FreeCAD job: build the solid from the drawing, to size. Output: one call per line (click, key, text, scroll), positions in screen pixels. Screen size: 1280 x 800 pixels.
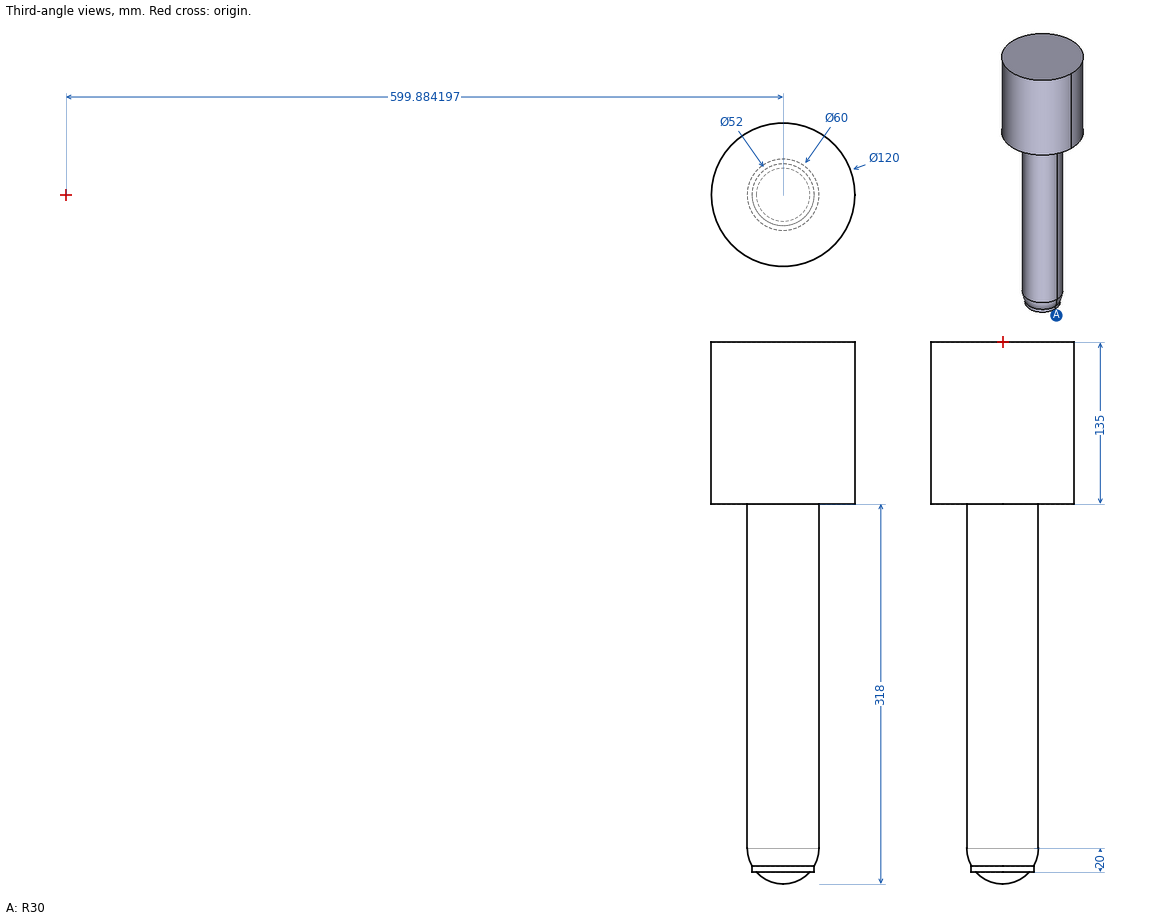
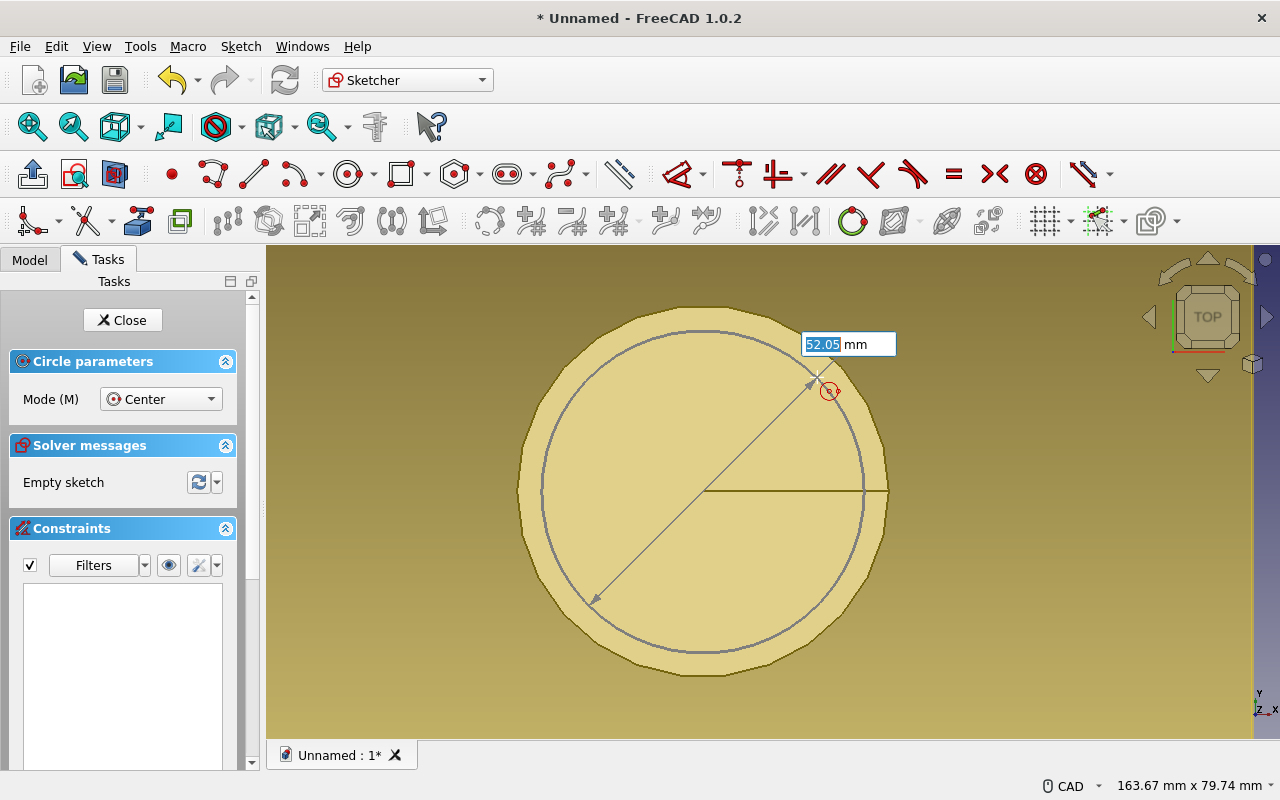
text(52)
key(Return)
key(Escape)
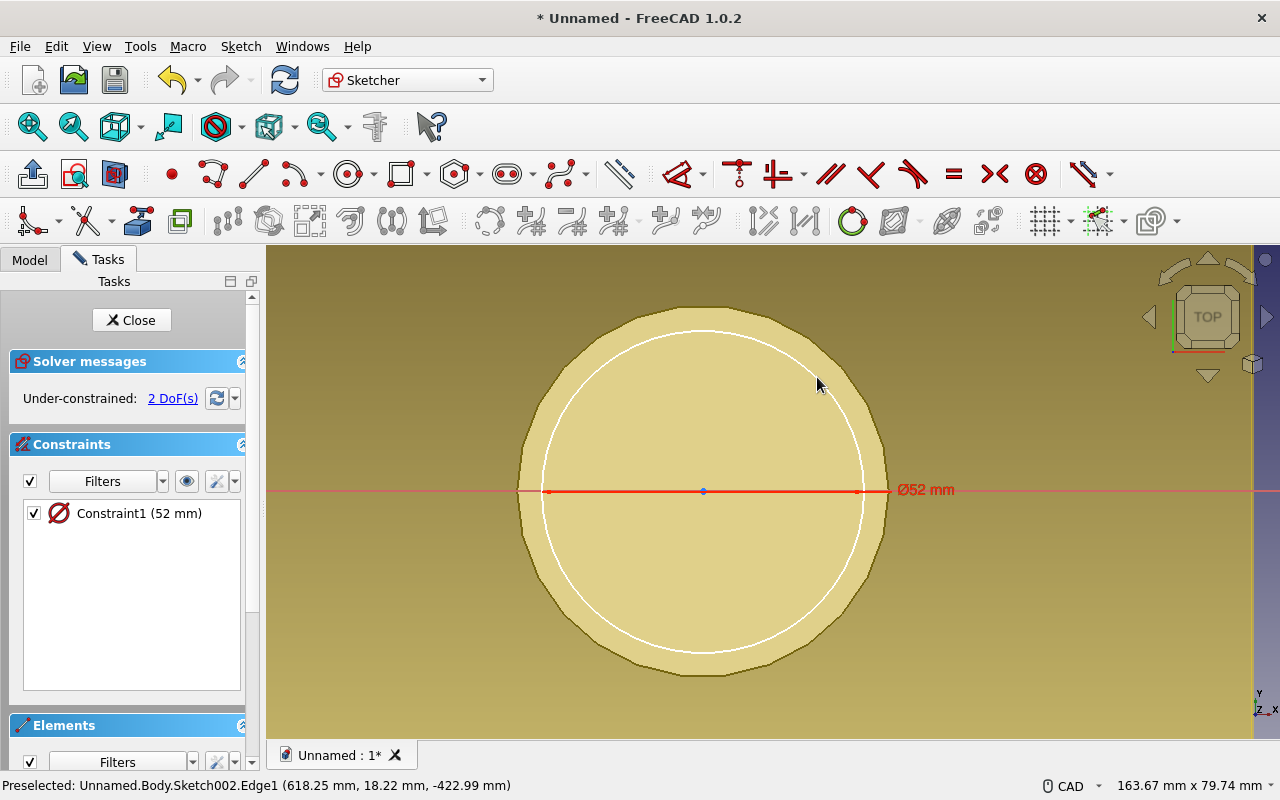
click(703, 492)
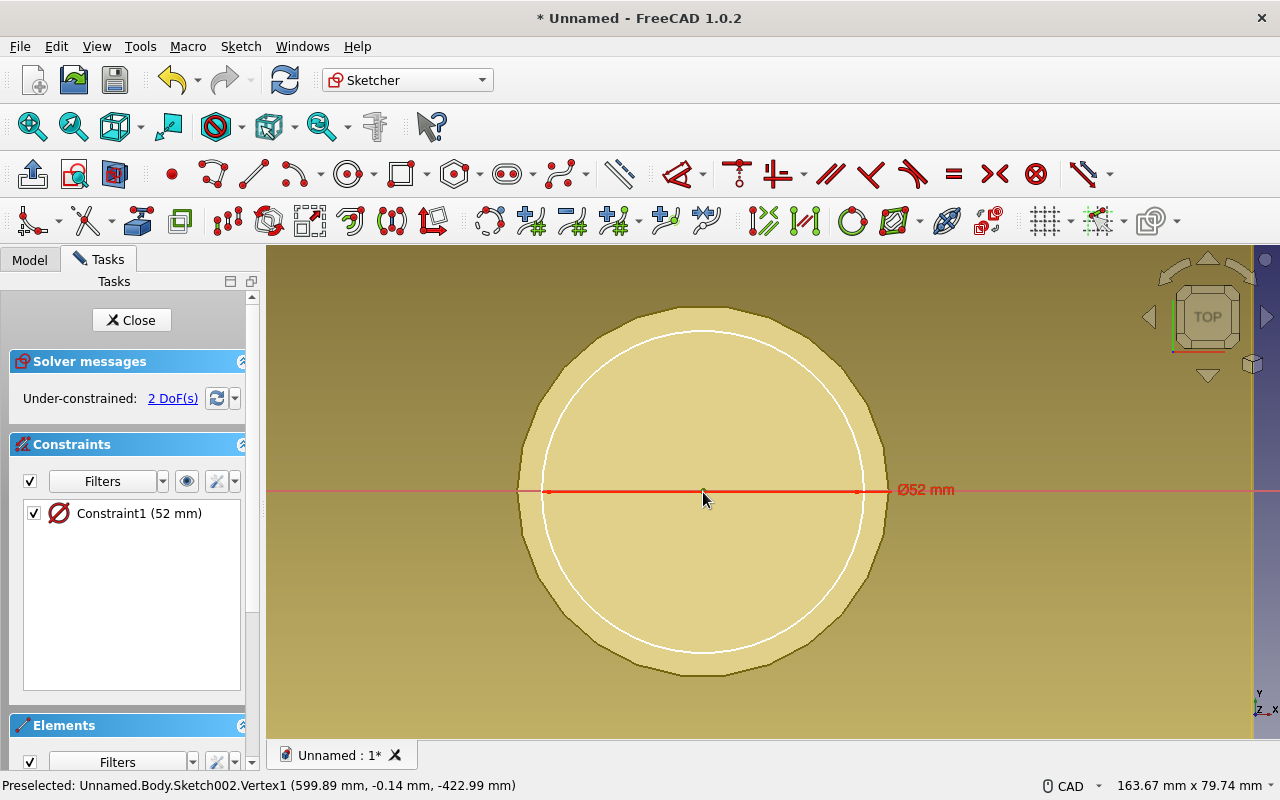
click(353, 491)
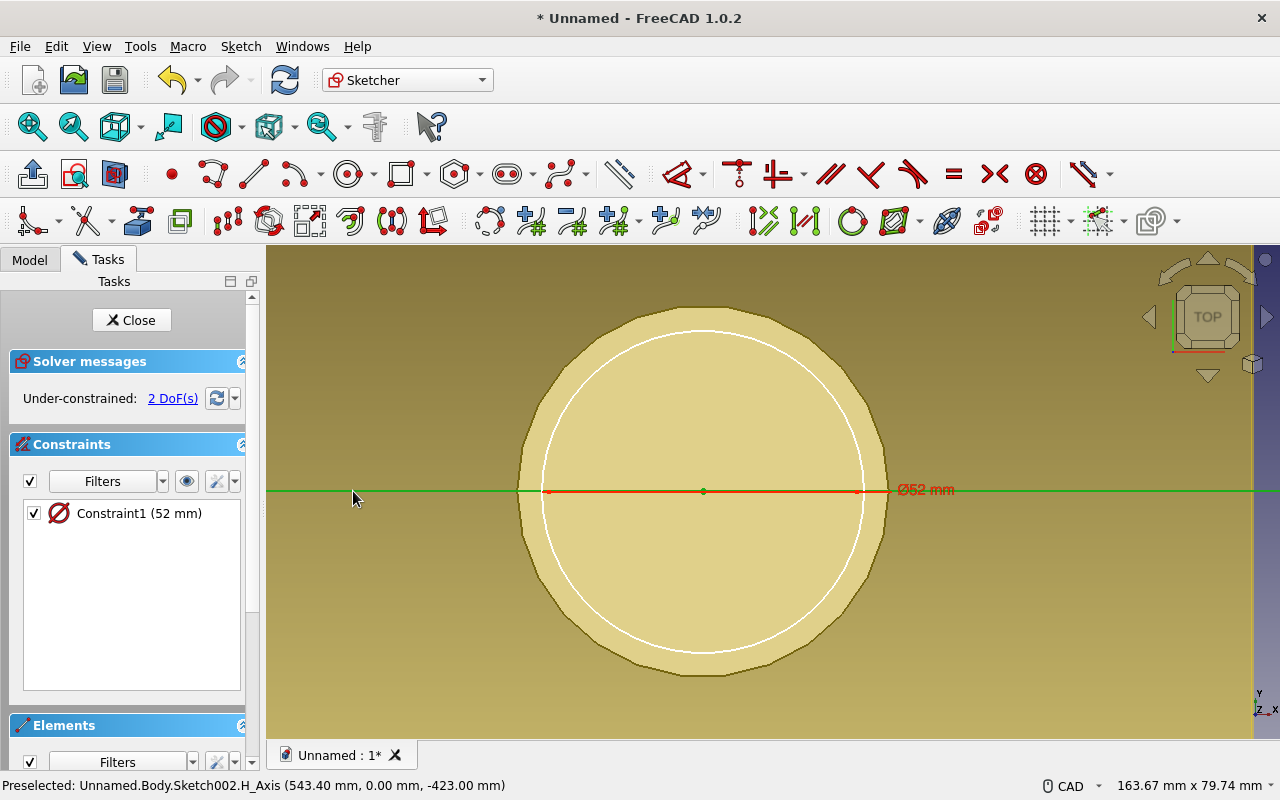
click(737, 174)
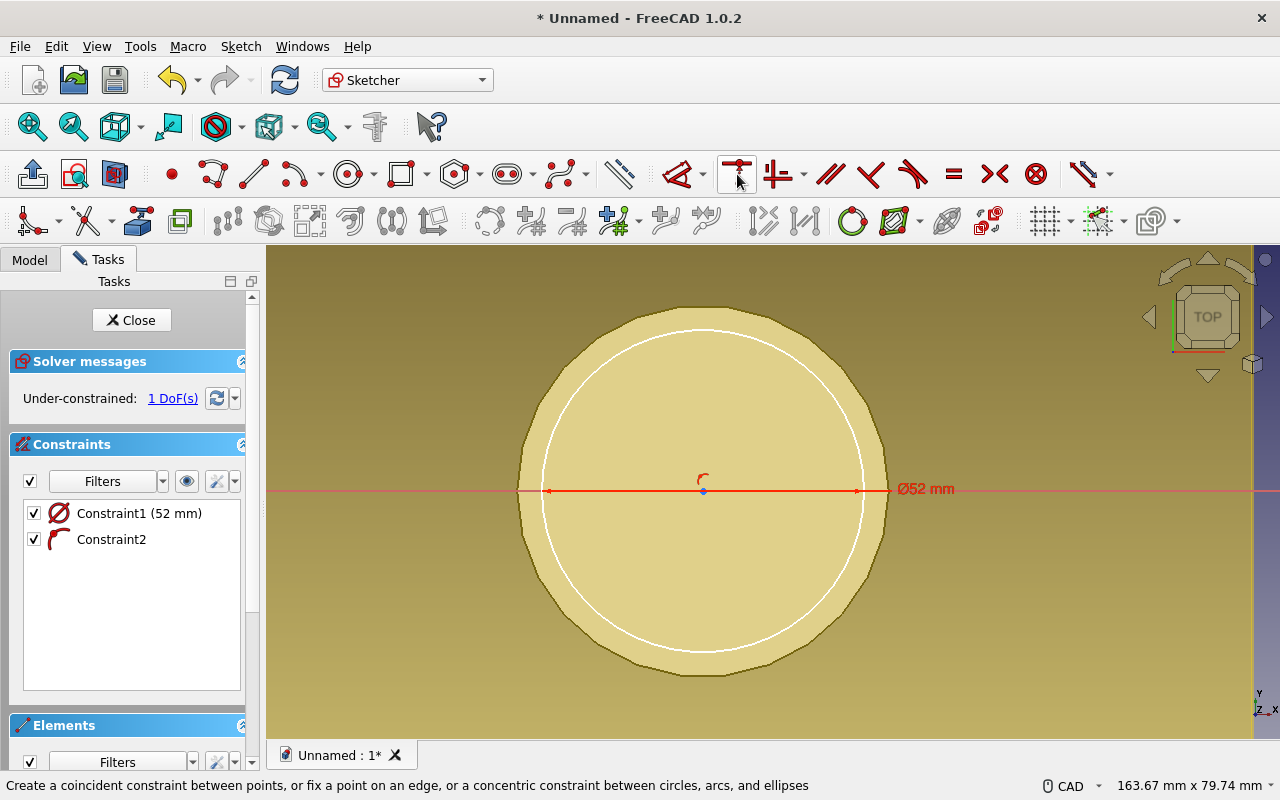
click(676, 174)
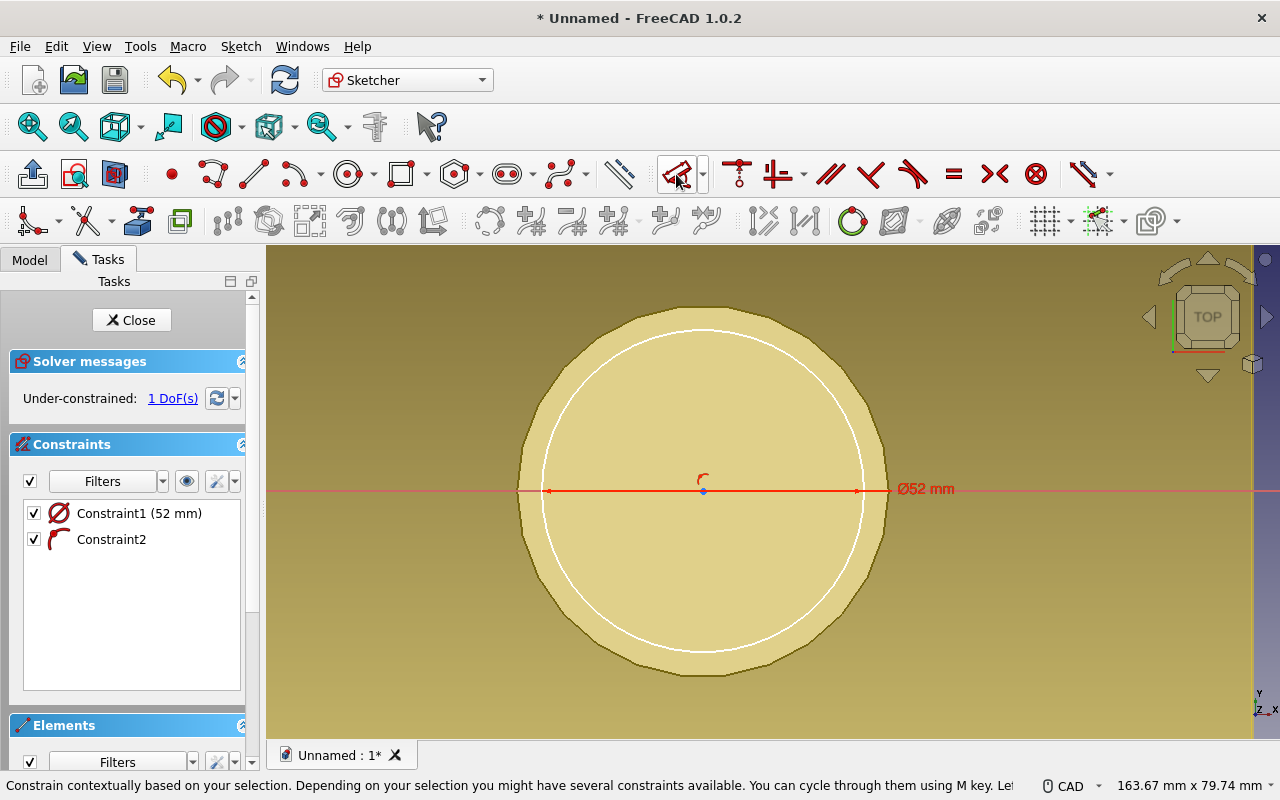
click(703, 491)
click(499, 525)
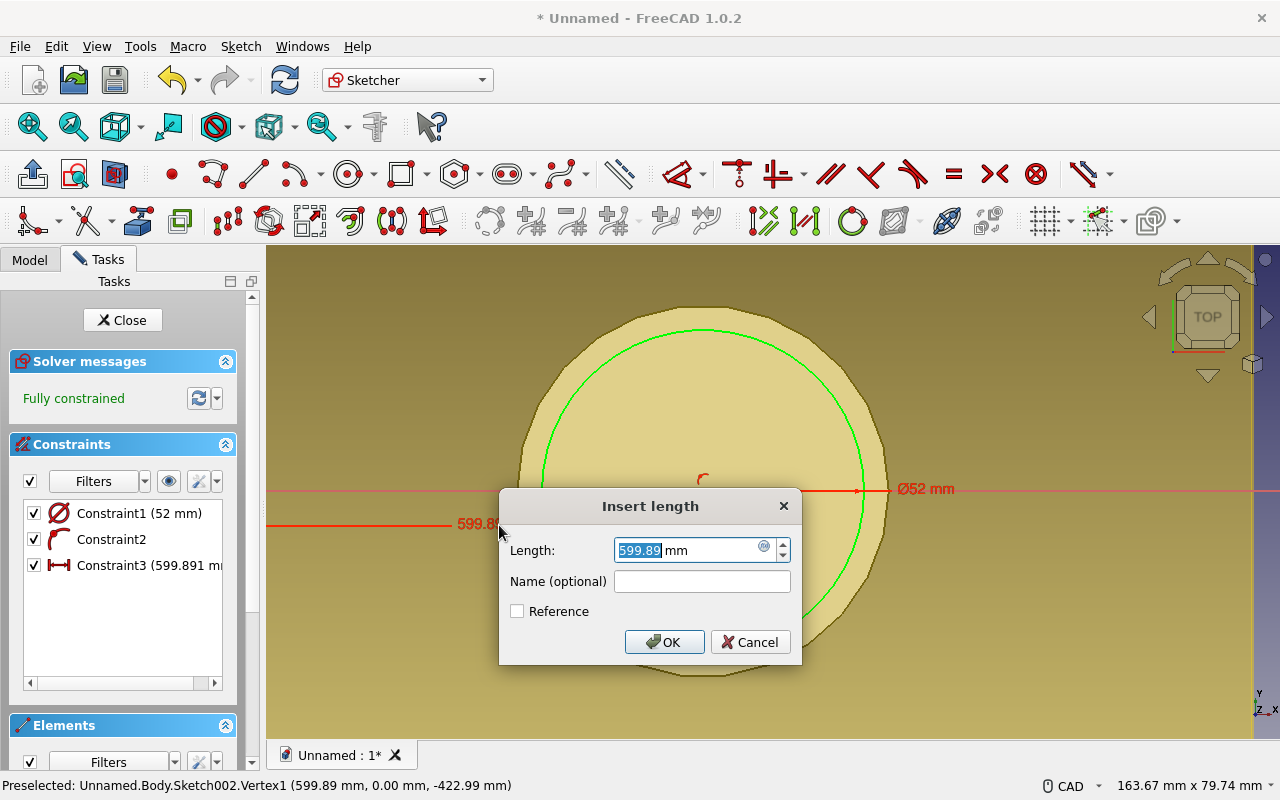
text(599.884197)
key(Return)
key(Escape)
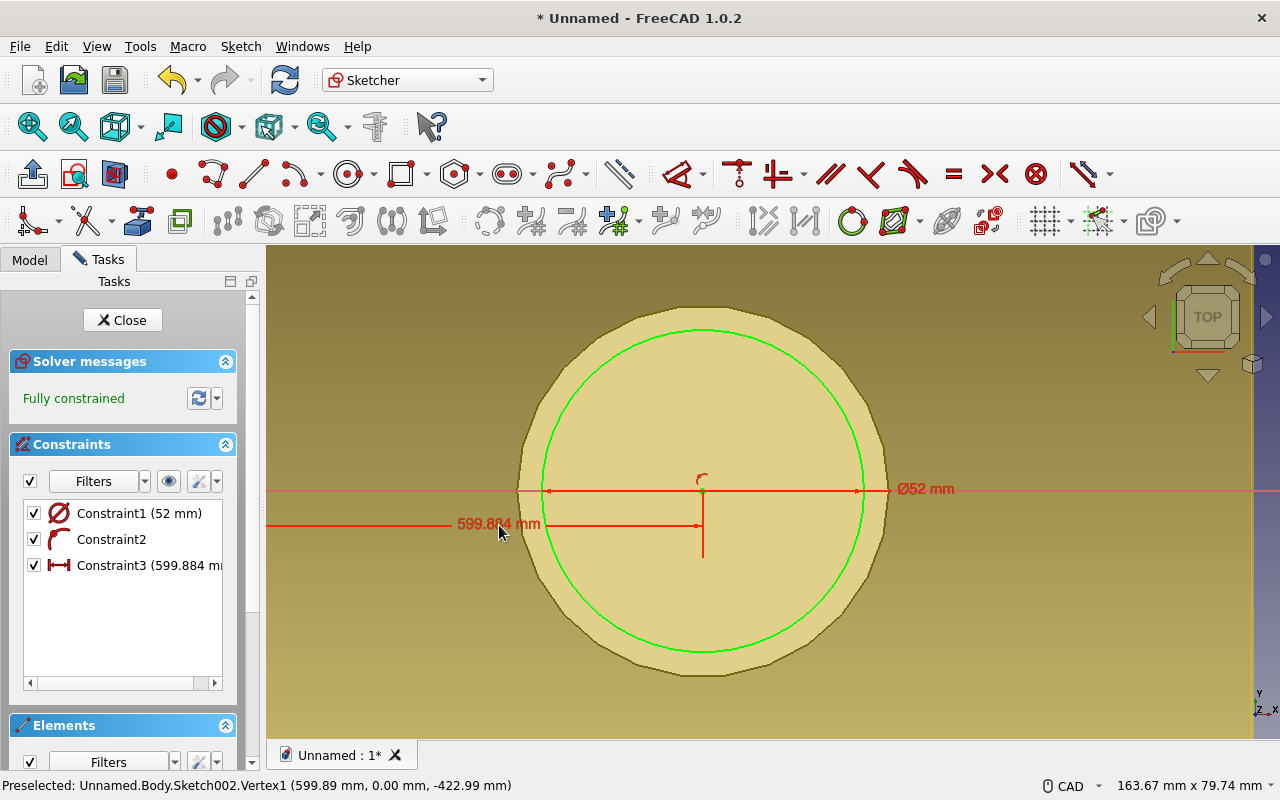
click(123, 320)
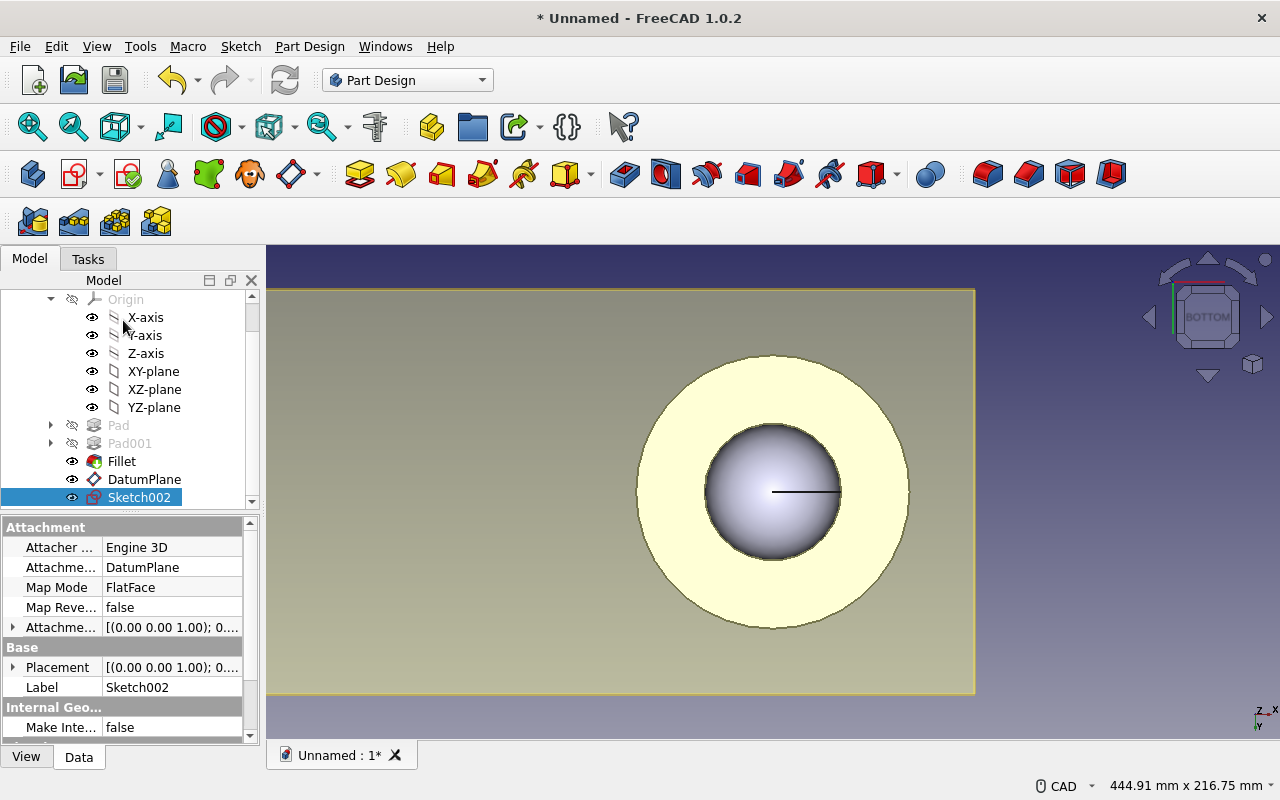
click(360, 174)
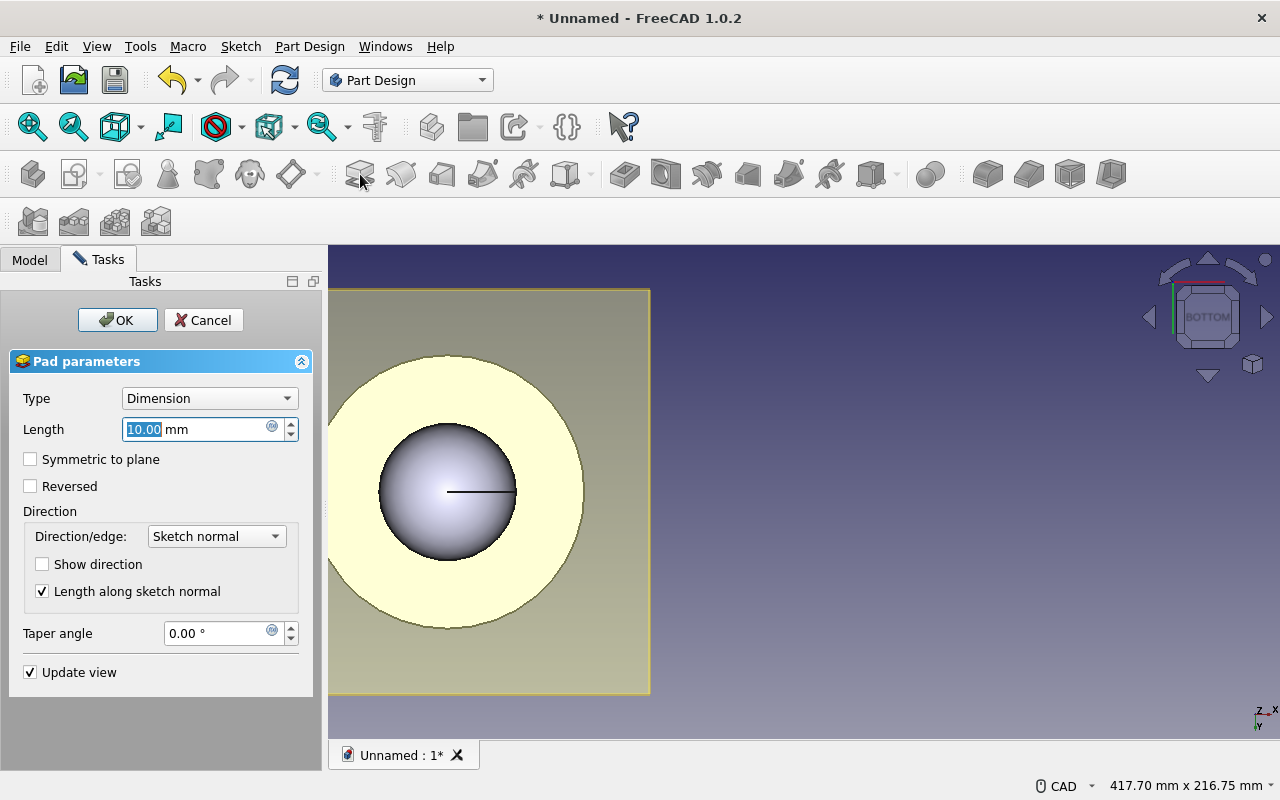
text(20)
key(Tab)